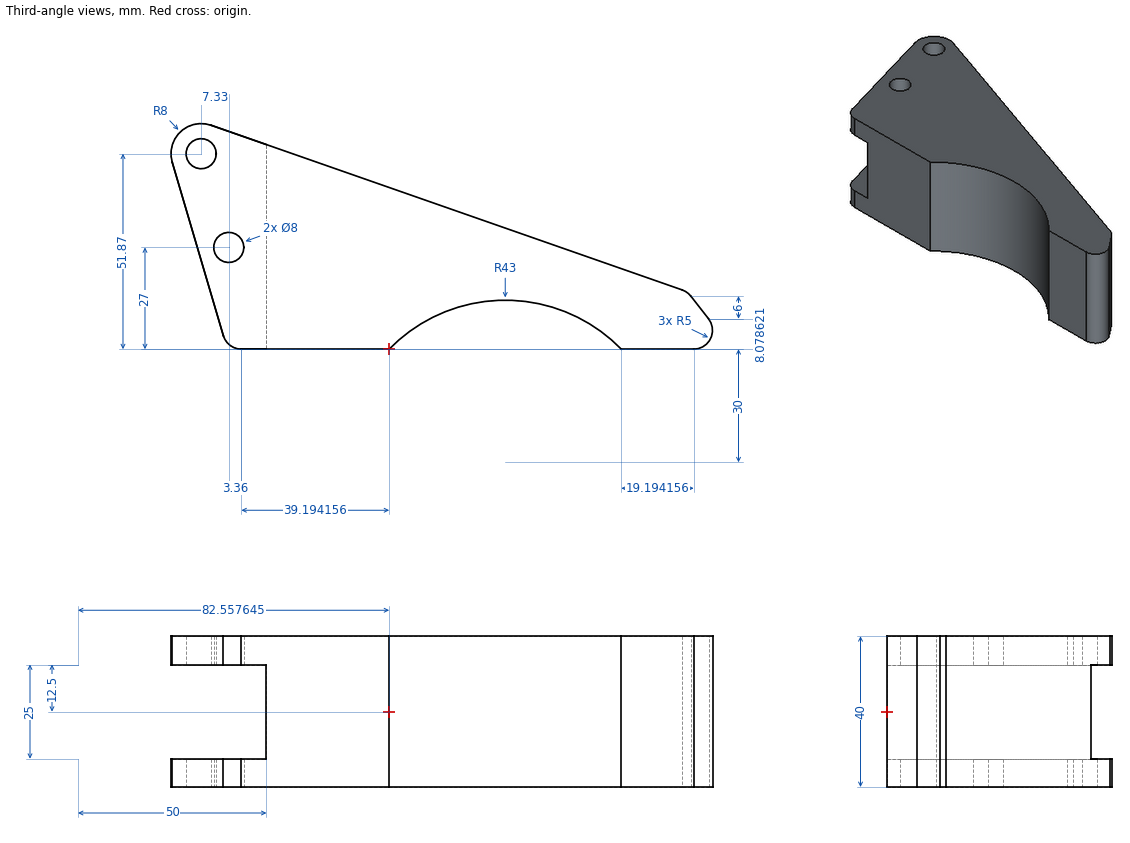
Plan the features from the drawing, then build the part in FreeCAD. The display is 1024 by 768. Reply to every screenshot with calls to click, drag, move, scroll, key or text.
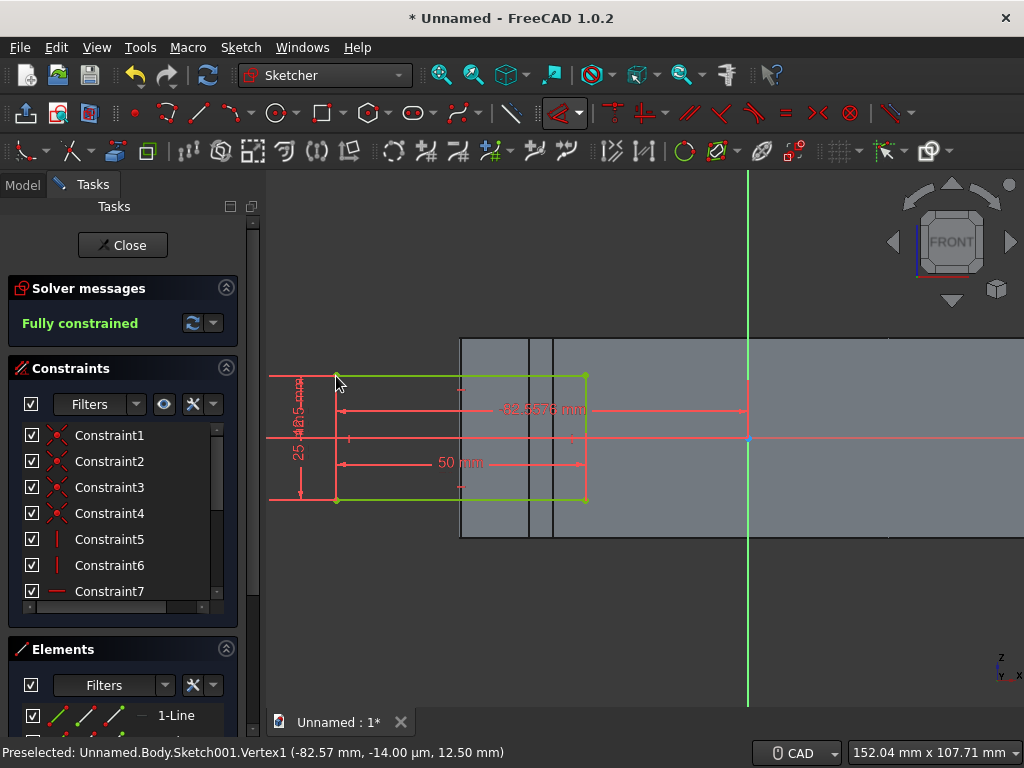
click(123, 245)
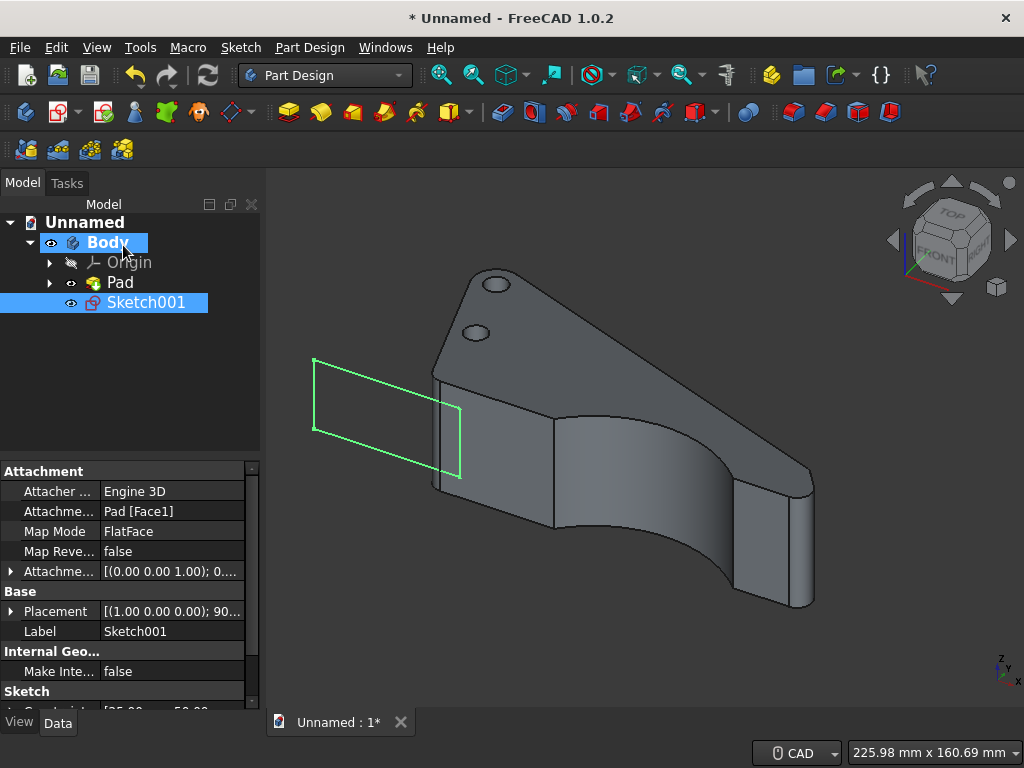
click(504, 112)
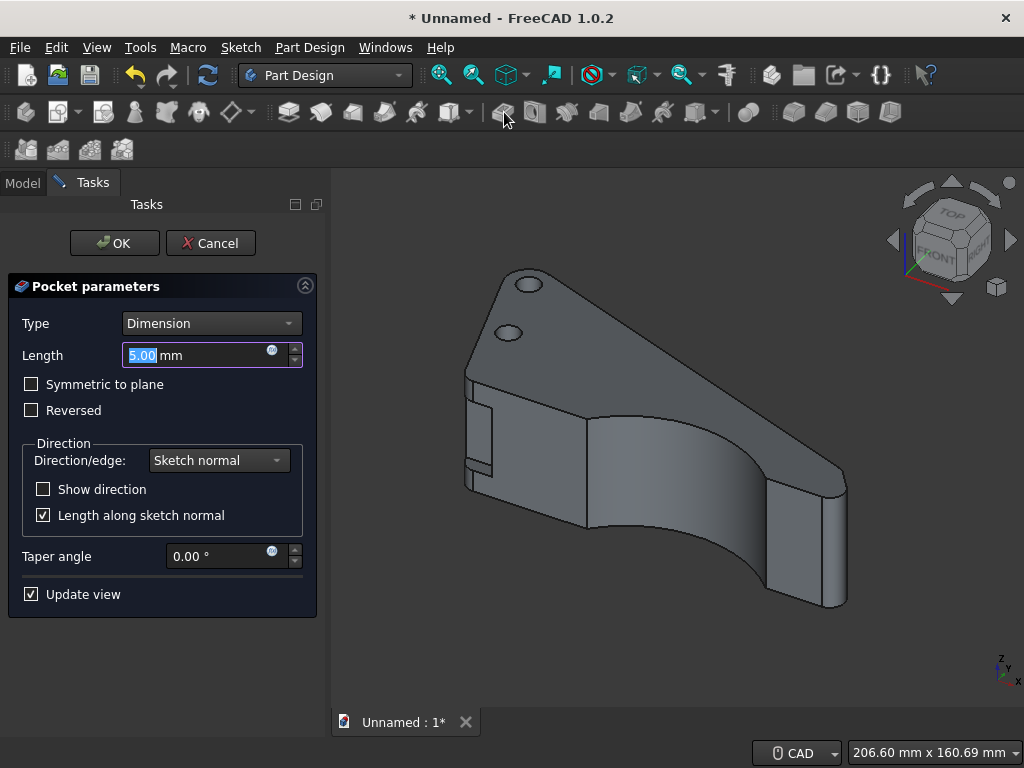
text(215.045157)
key(Tab)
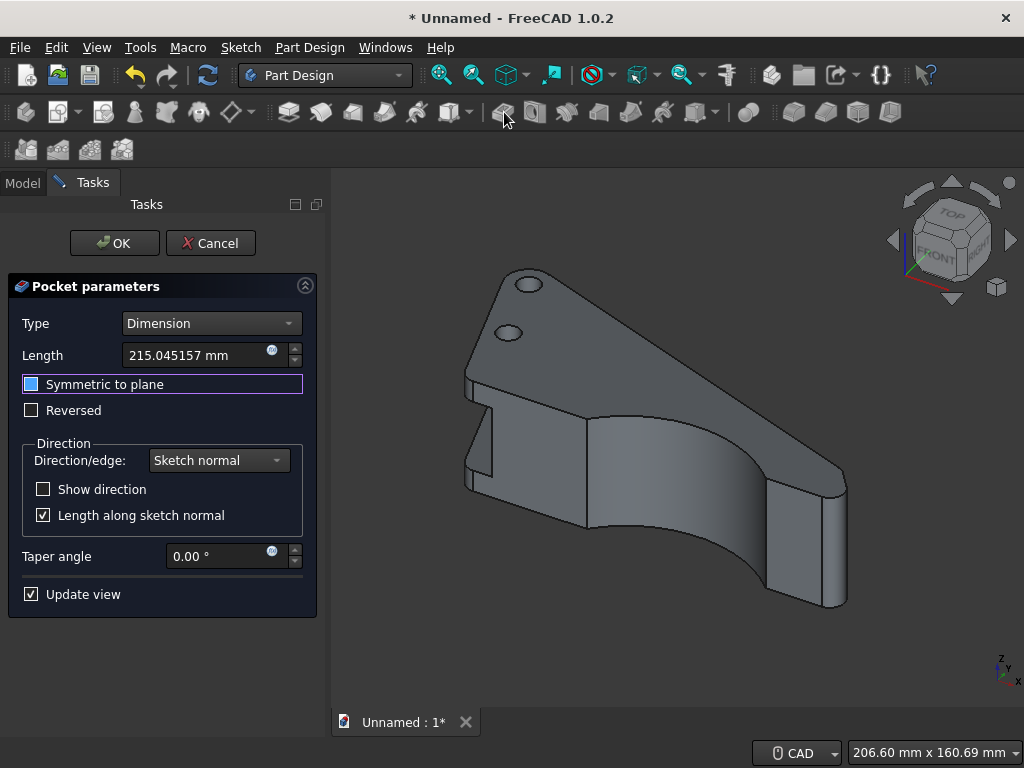
click(30, 384)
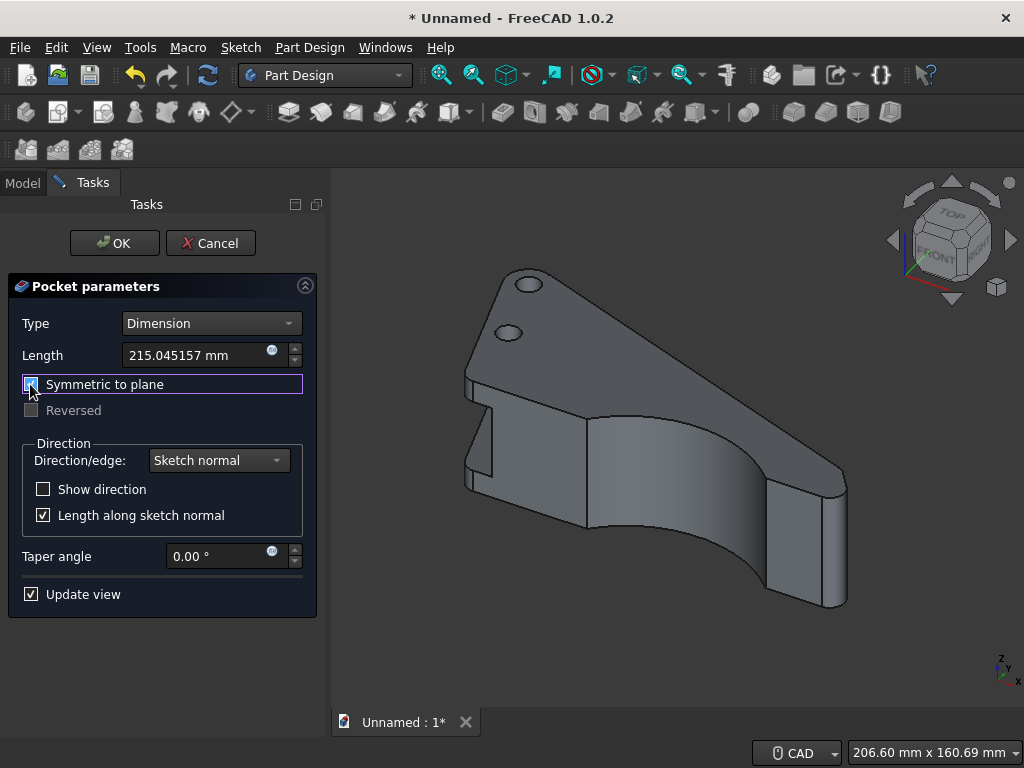
click(115, 243)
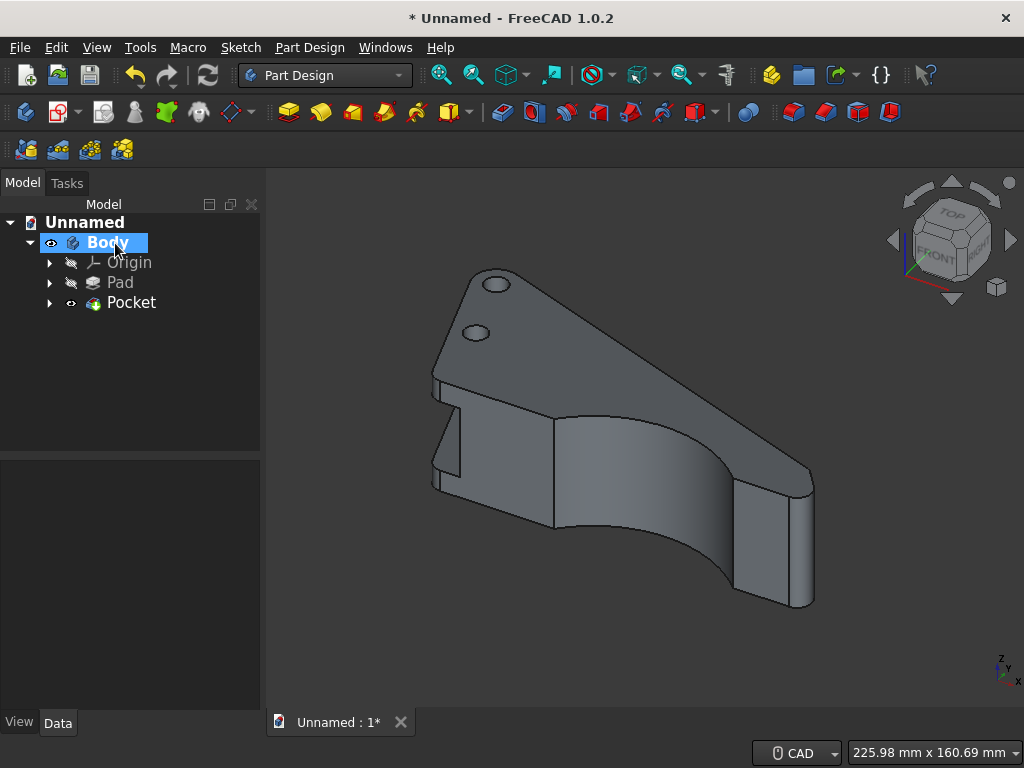
key(0)